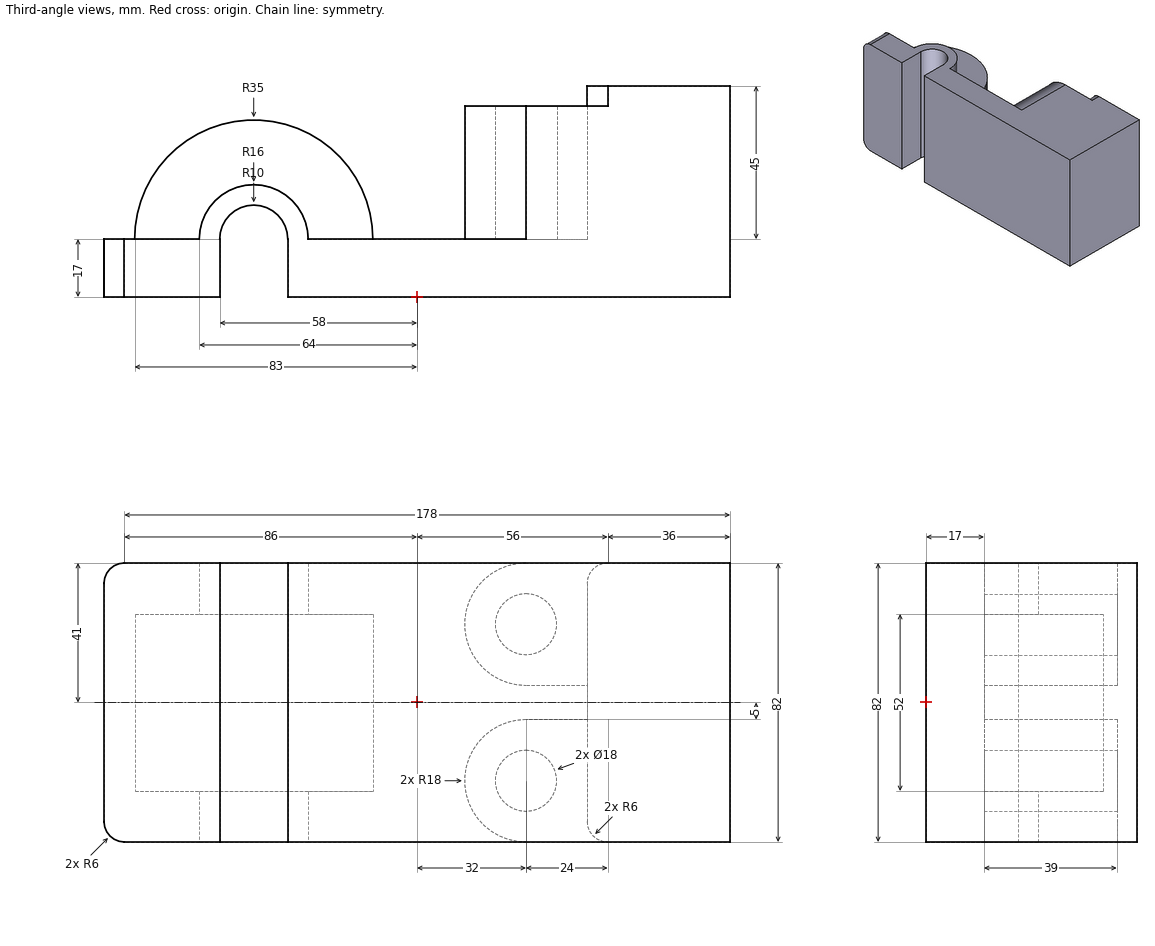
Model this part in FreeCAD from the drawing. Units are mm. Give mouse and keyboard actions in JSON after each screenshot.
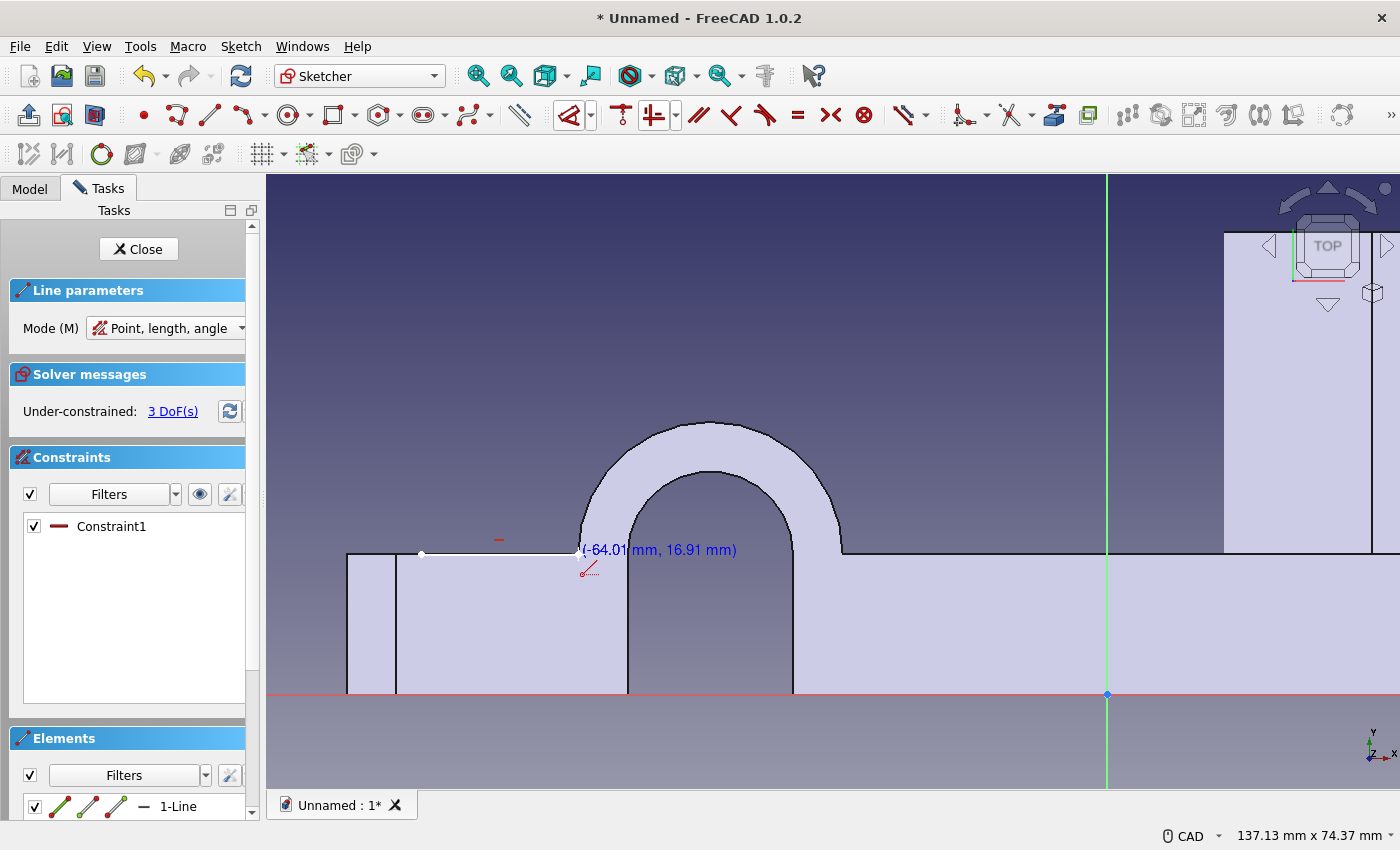
{"action": "left_click", "coordinate": [843, 554]}
{"action": "left_click", "coordinate": [1000, 554]}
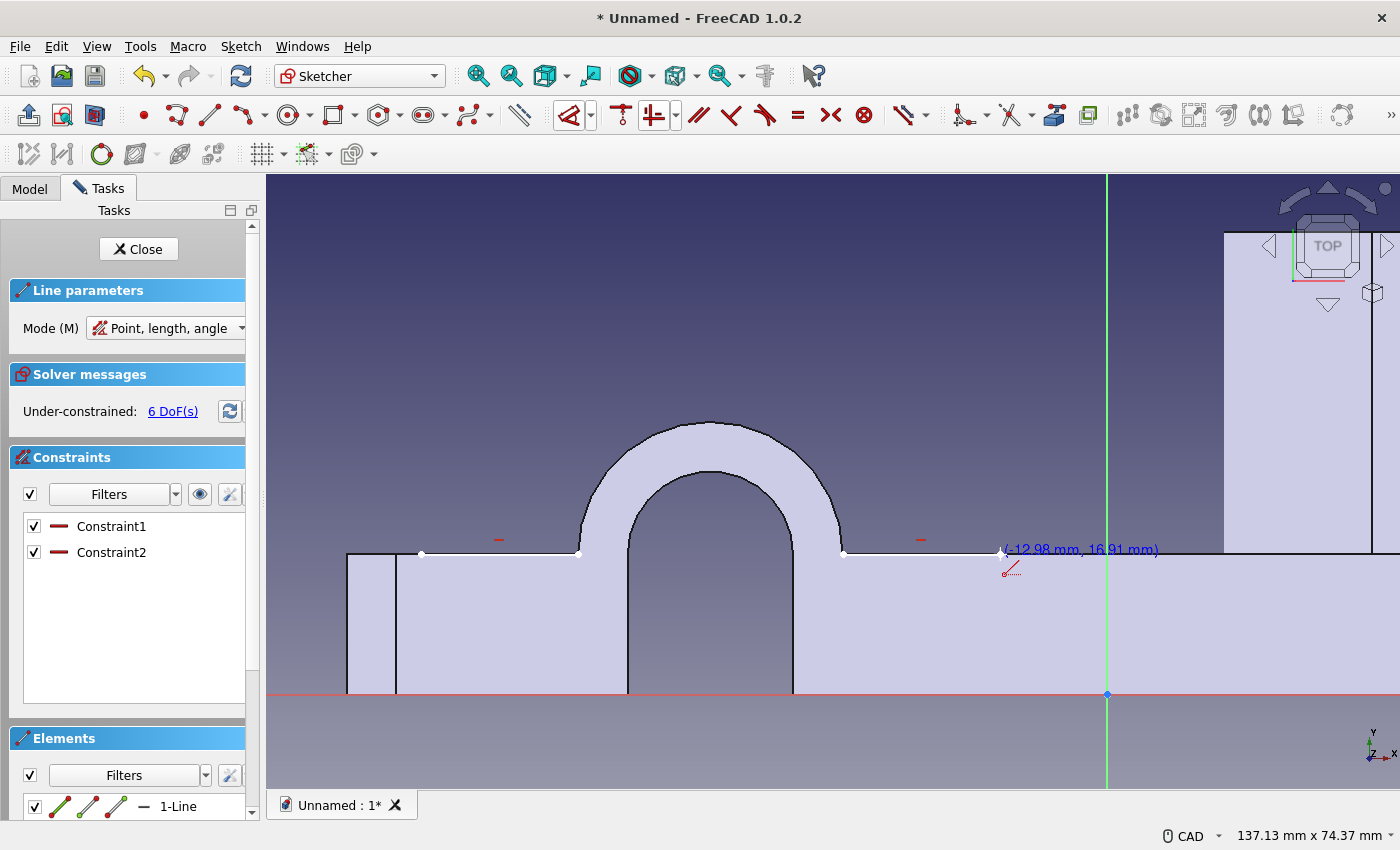
{"action": "left_click", "coordinate": [242, 116]}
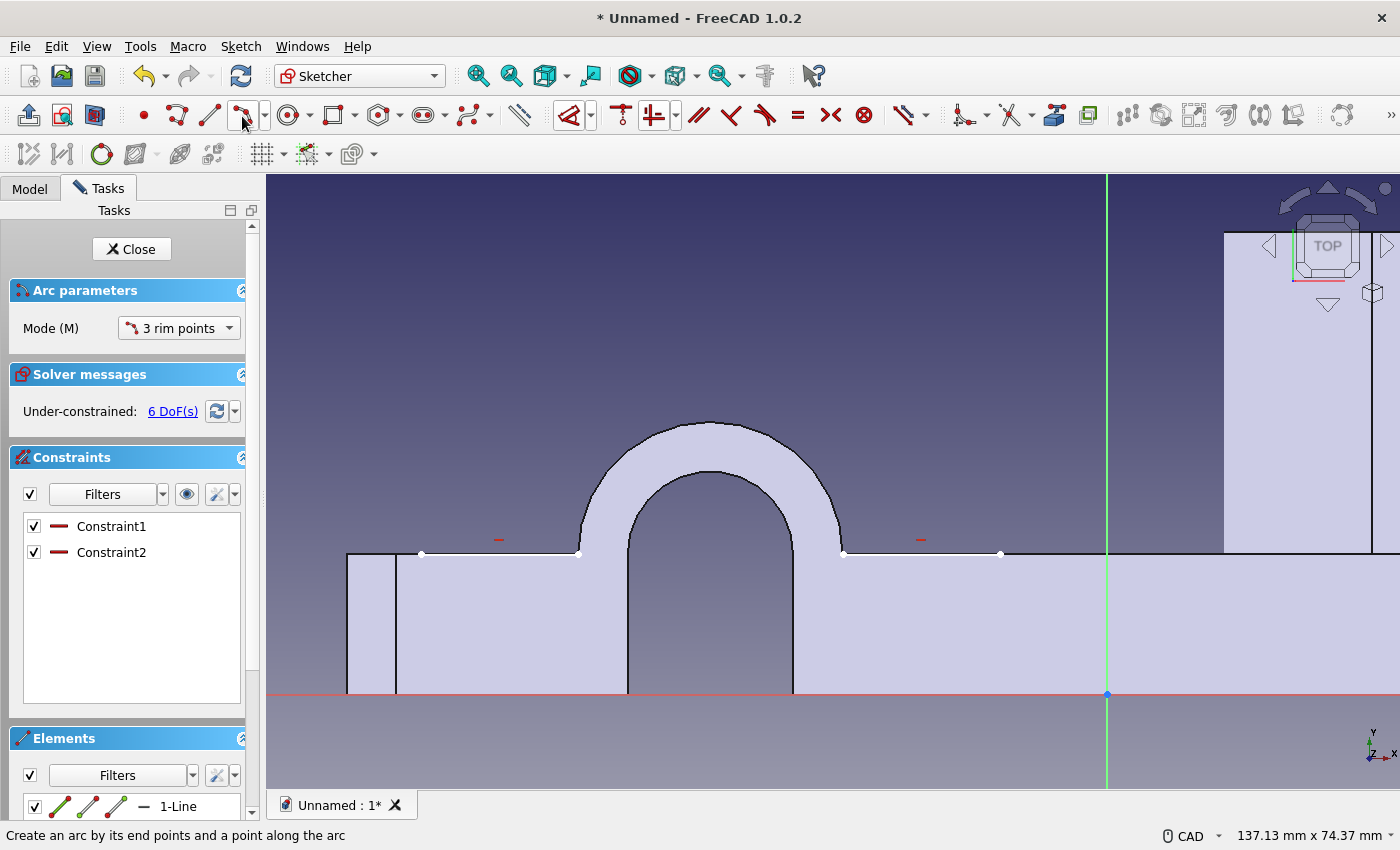
{"action": "left_click", "coordinate": [578, 555]}
{"action": "left_click", "coordinate": [843, 555]}
{"action": "left_click", "coordinate": [710, 422]}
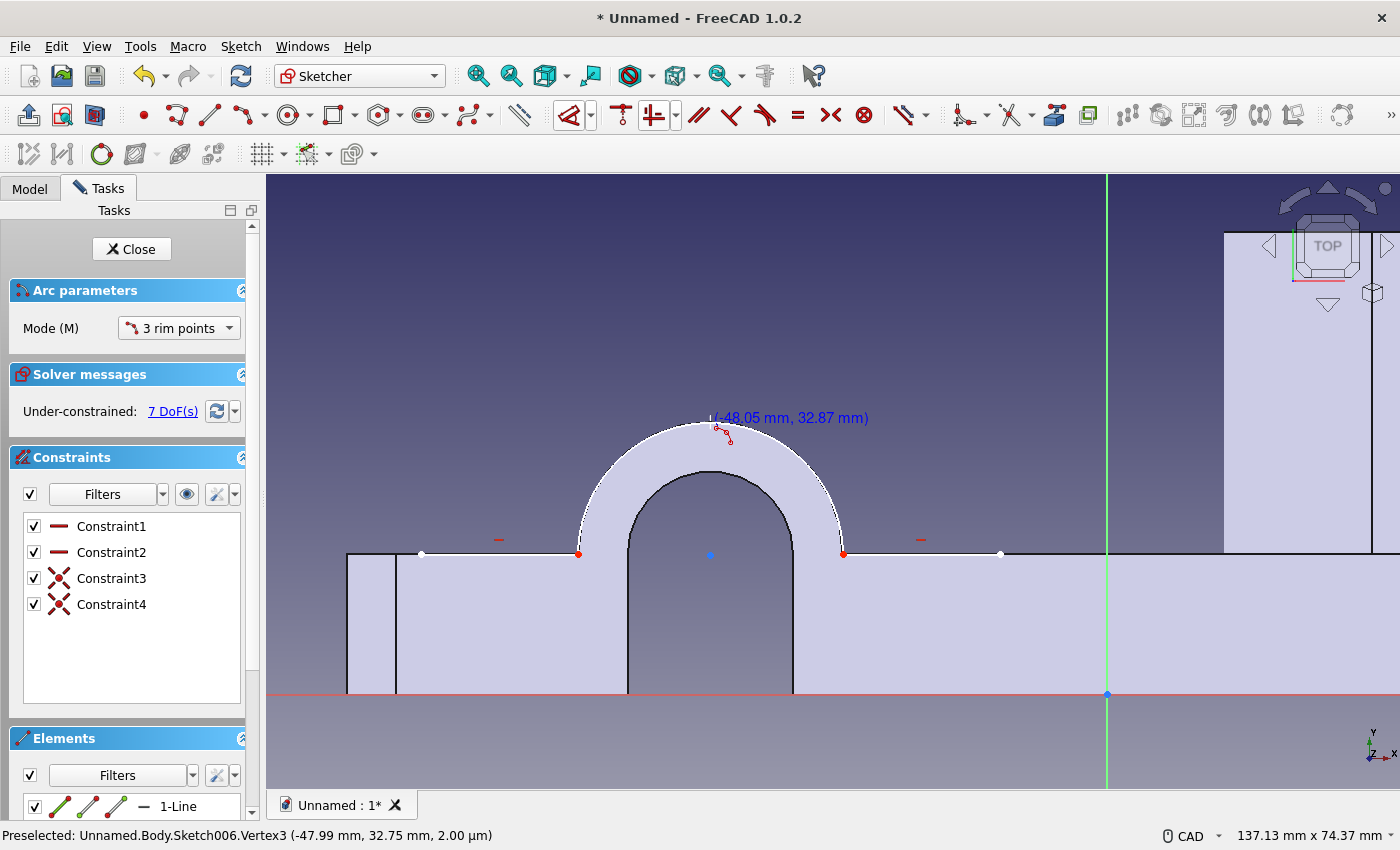
{"action": "left_click", "coordinate": [1000, 555]}
{"action": "left_click", "coordinate": [421, 555]}
{"action": "left_click", "coordinate": [710, 265]}
{"action": "key", "text": "Escape"}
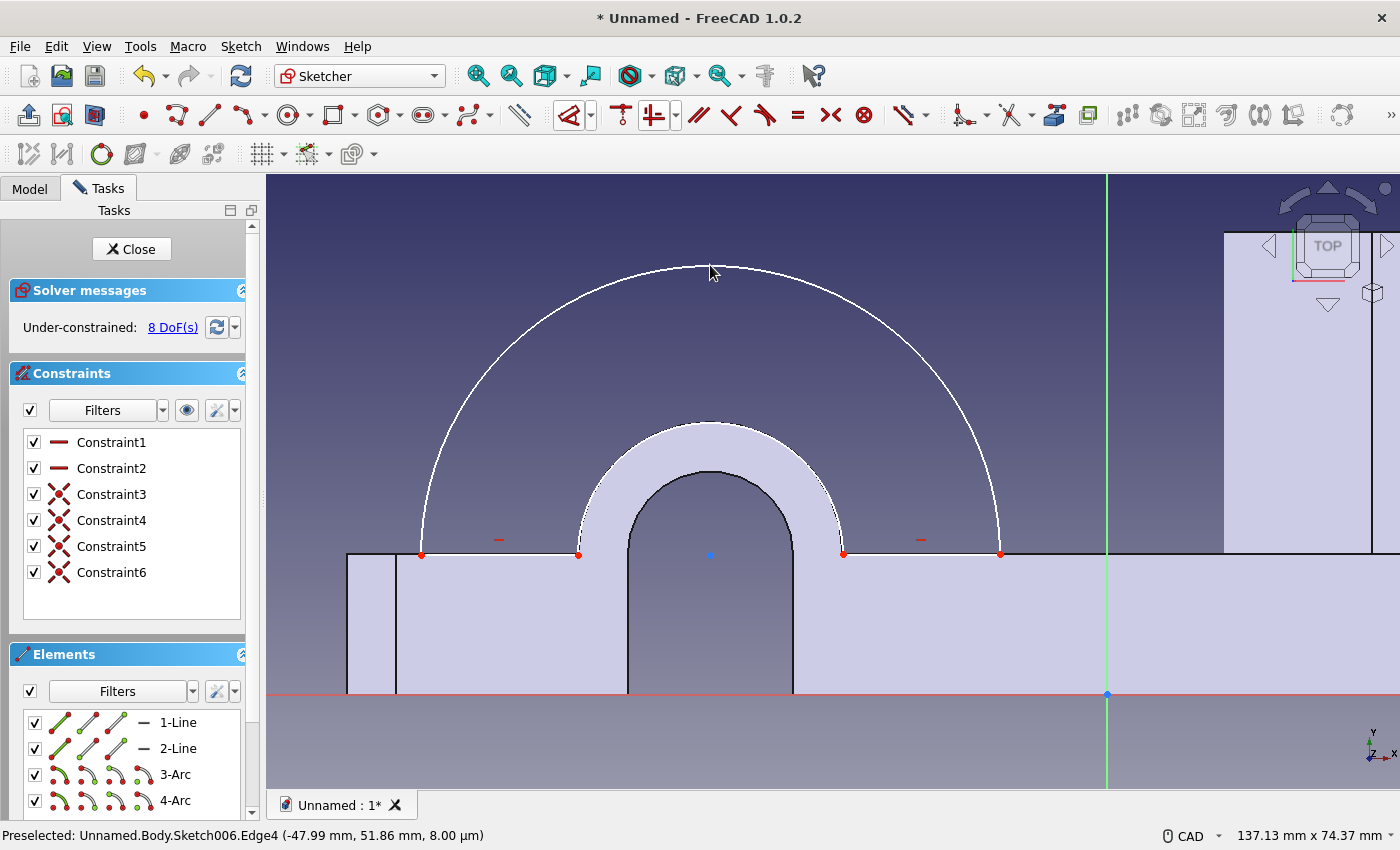
{"action": "left_click", "coordinate": [788, 448]}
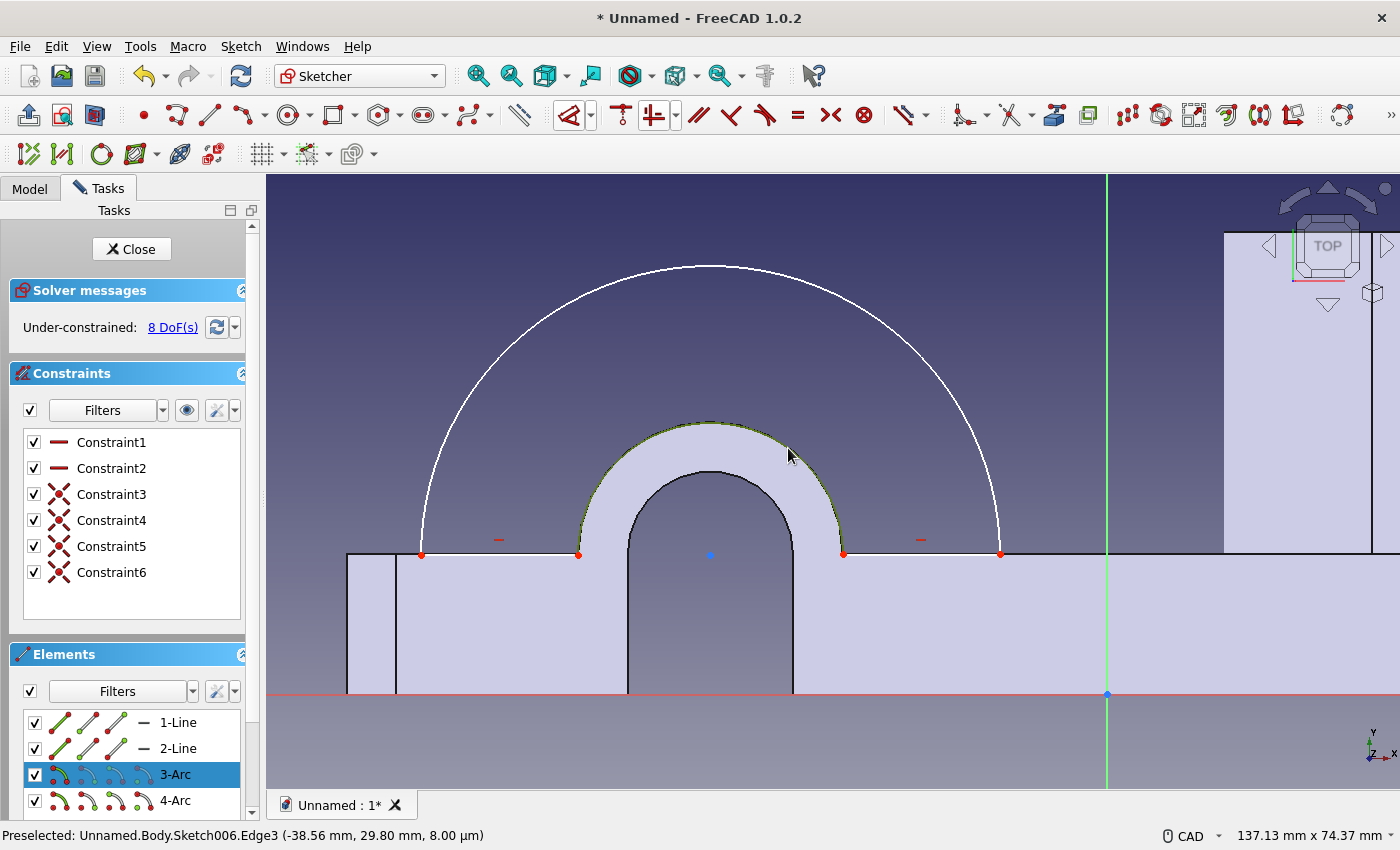
{"action": "left_click", "coordinate": [881, 321]}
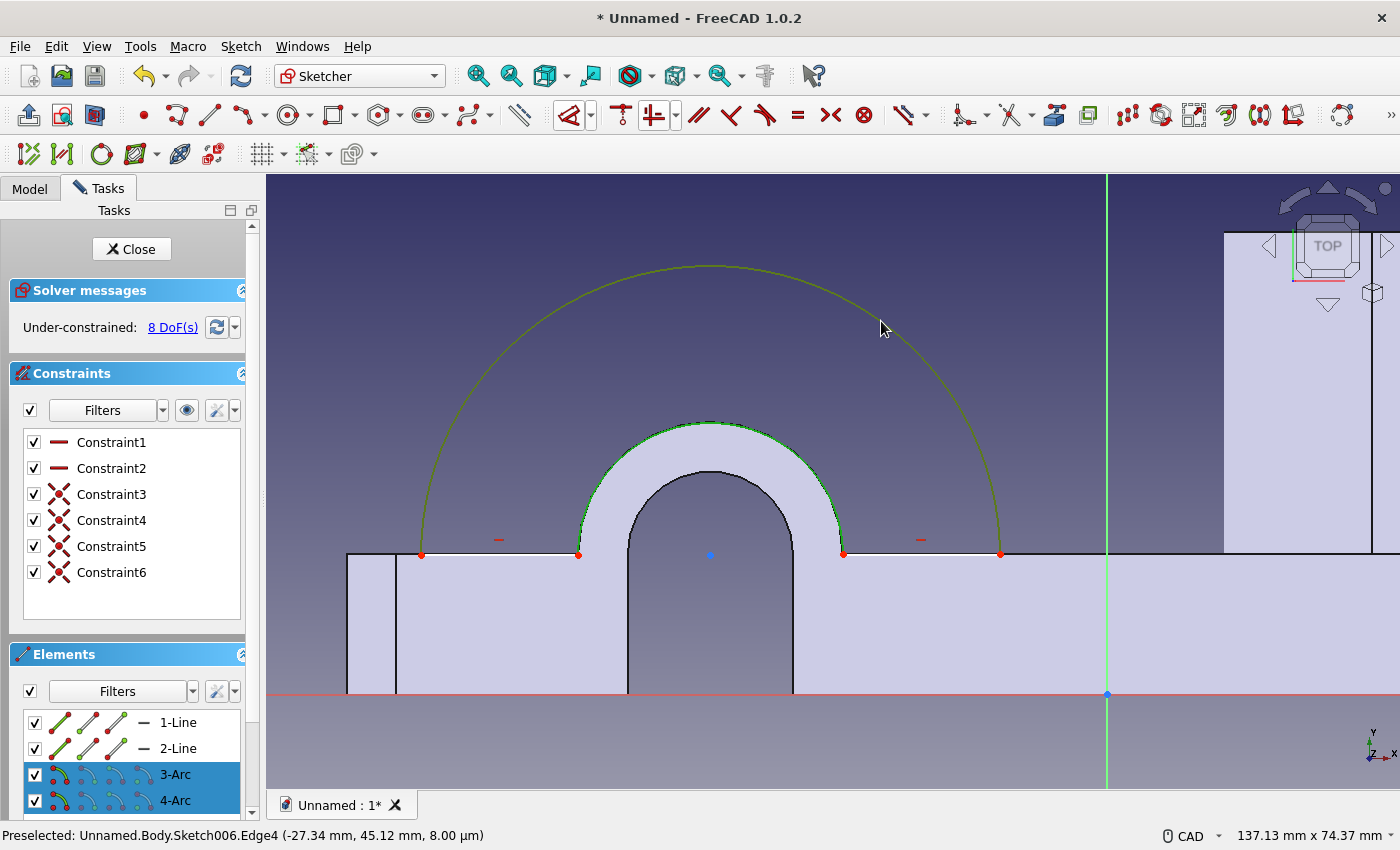
{"action": "left_click", "coordinate": [621, 116]}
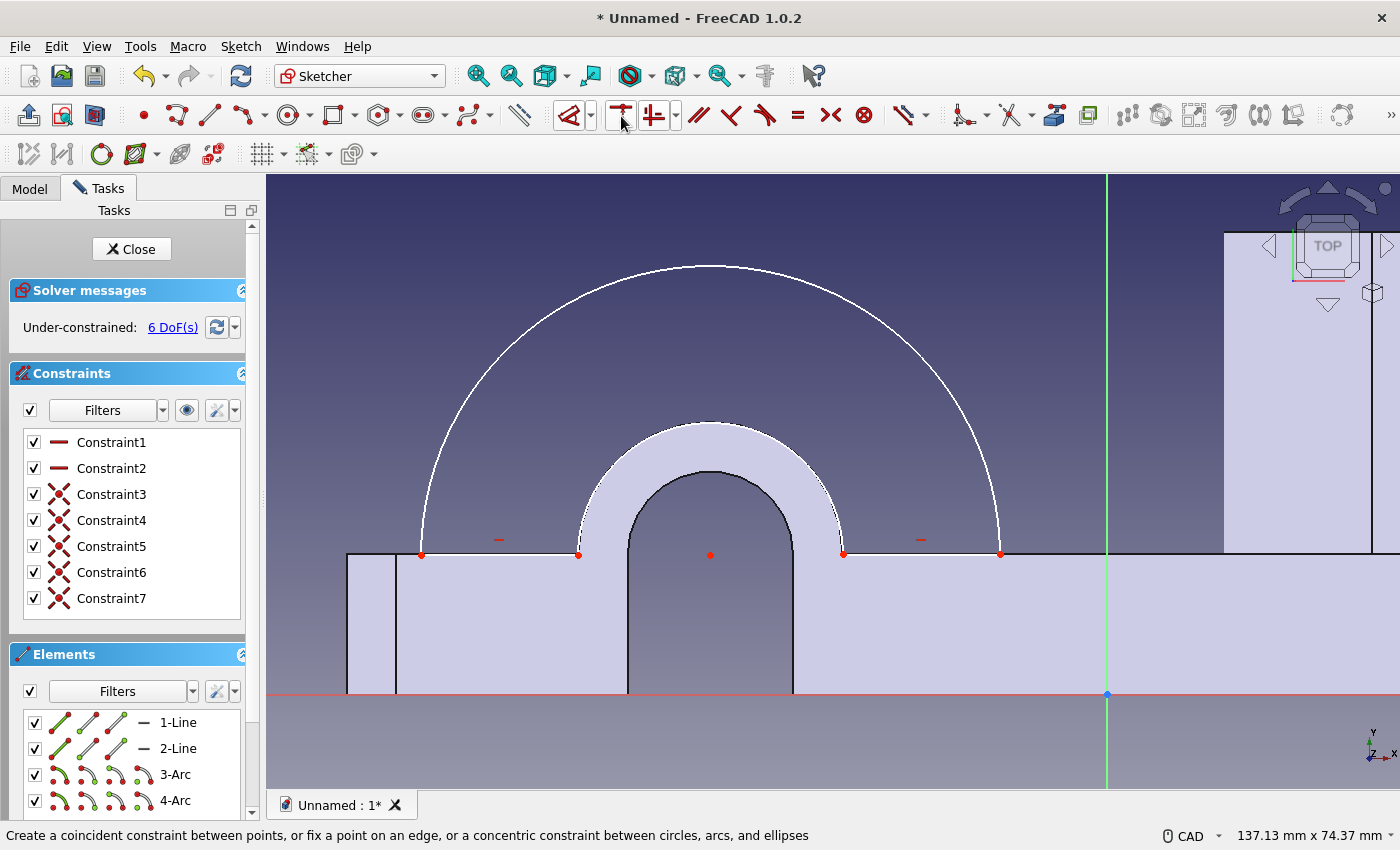
{"action": "left_click", "coordinate": [788, 448]}